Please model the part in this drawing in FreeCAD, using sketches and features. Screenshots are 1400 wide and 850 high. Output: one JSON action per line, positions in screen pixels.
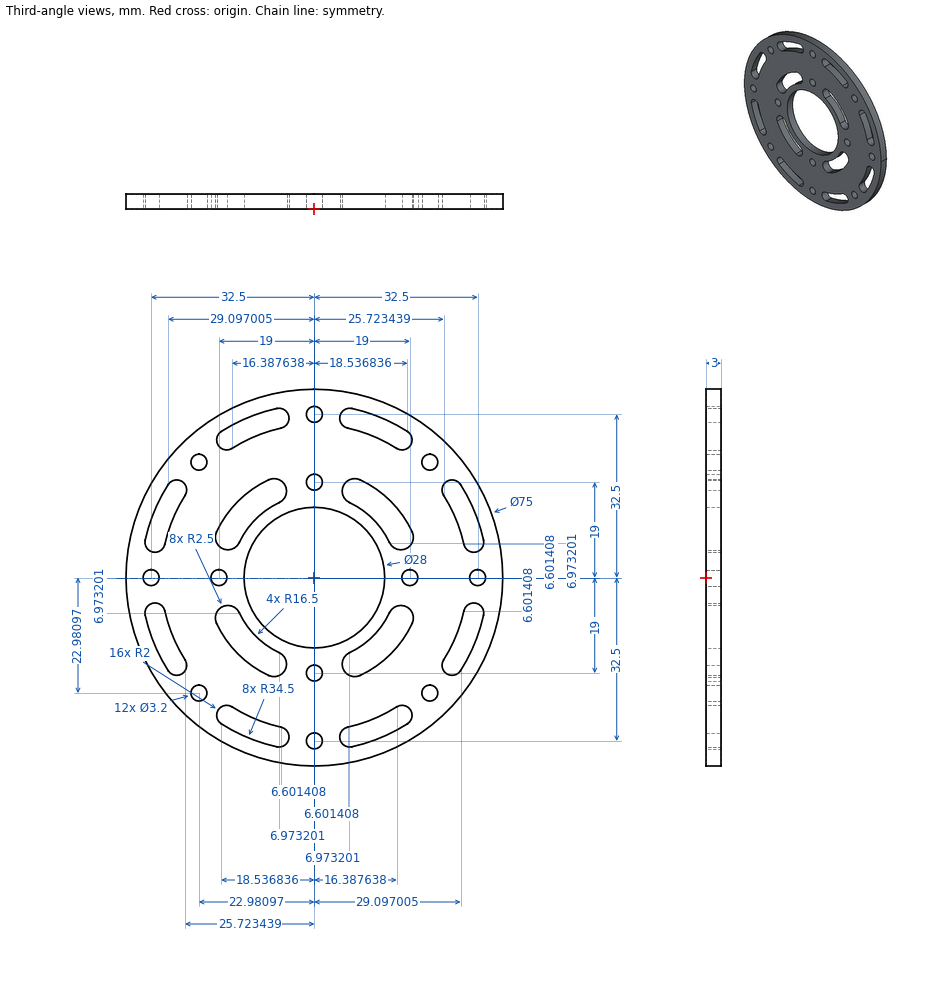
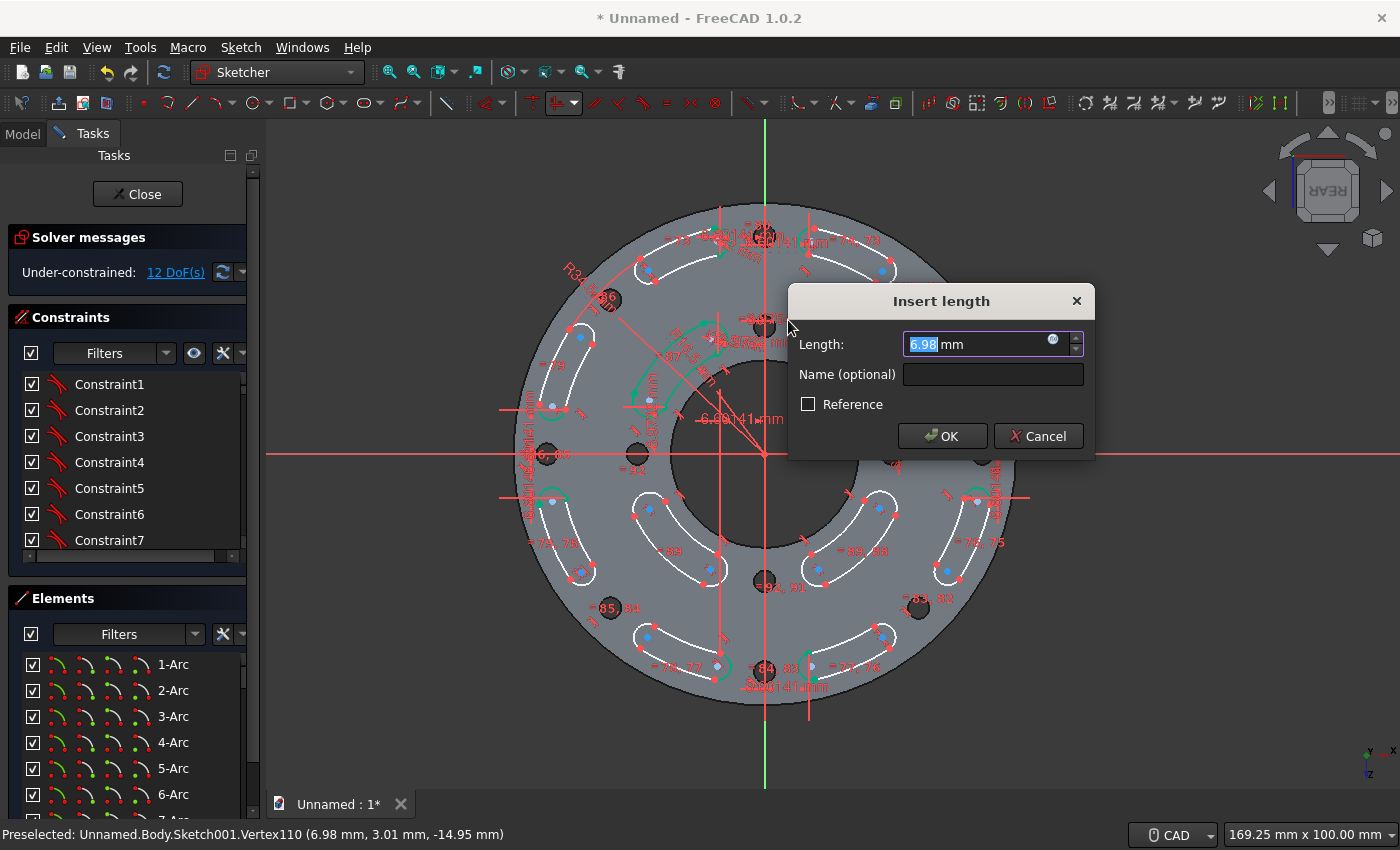
{"action": "type", "text": "6.973201"}
{"action": "key", "text": "Return"}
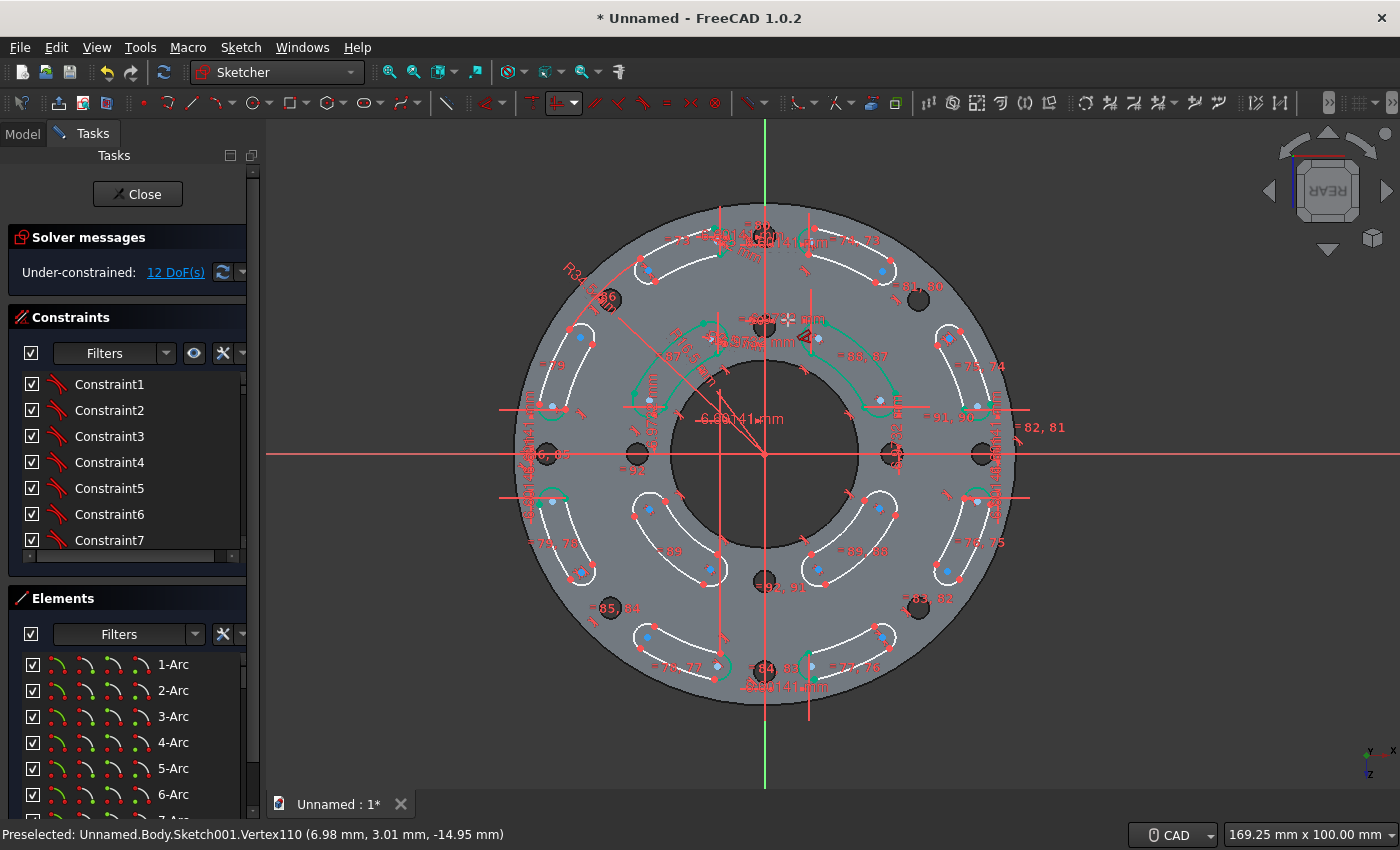
{"action": "left_click", "coordinate": [811, 554]}
{"action": "left_click", "coordinate": [788, 588]}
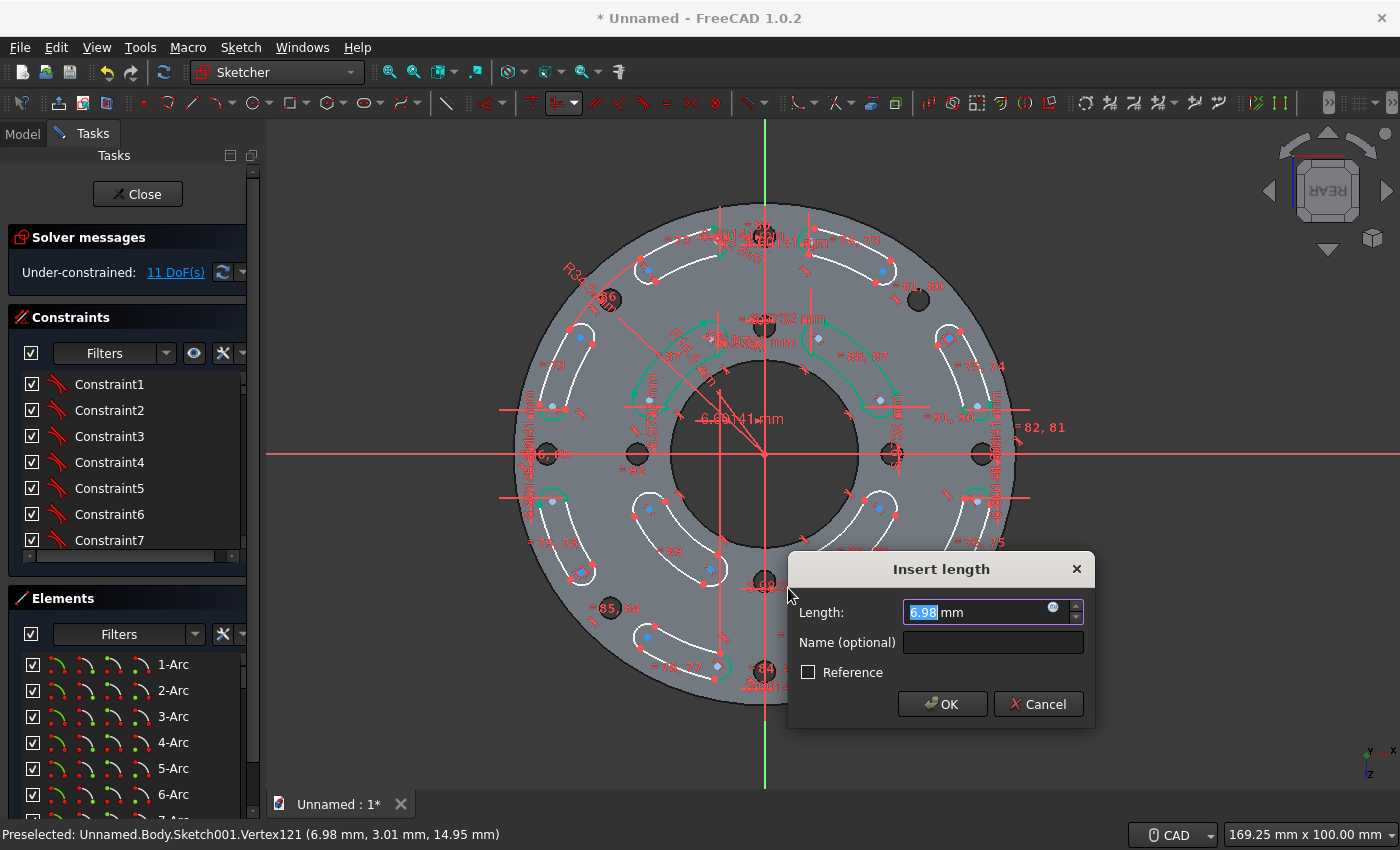
{"action": "type", "text": "6.973201"}
{"action": "key", "text": "Return"}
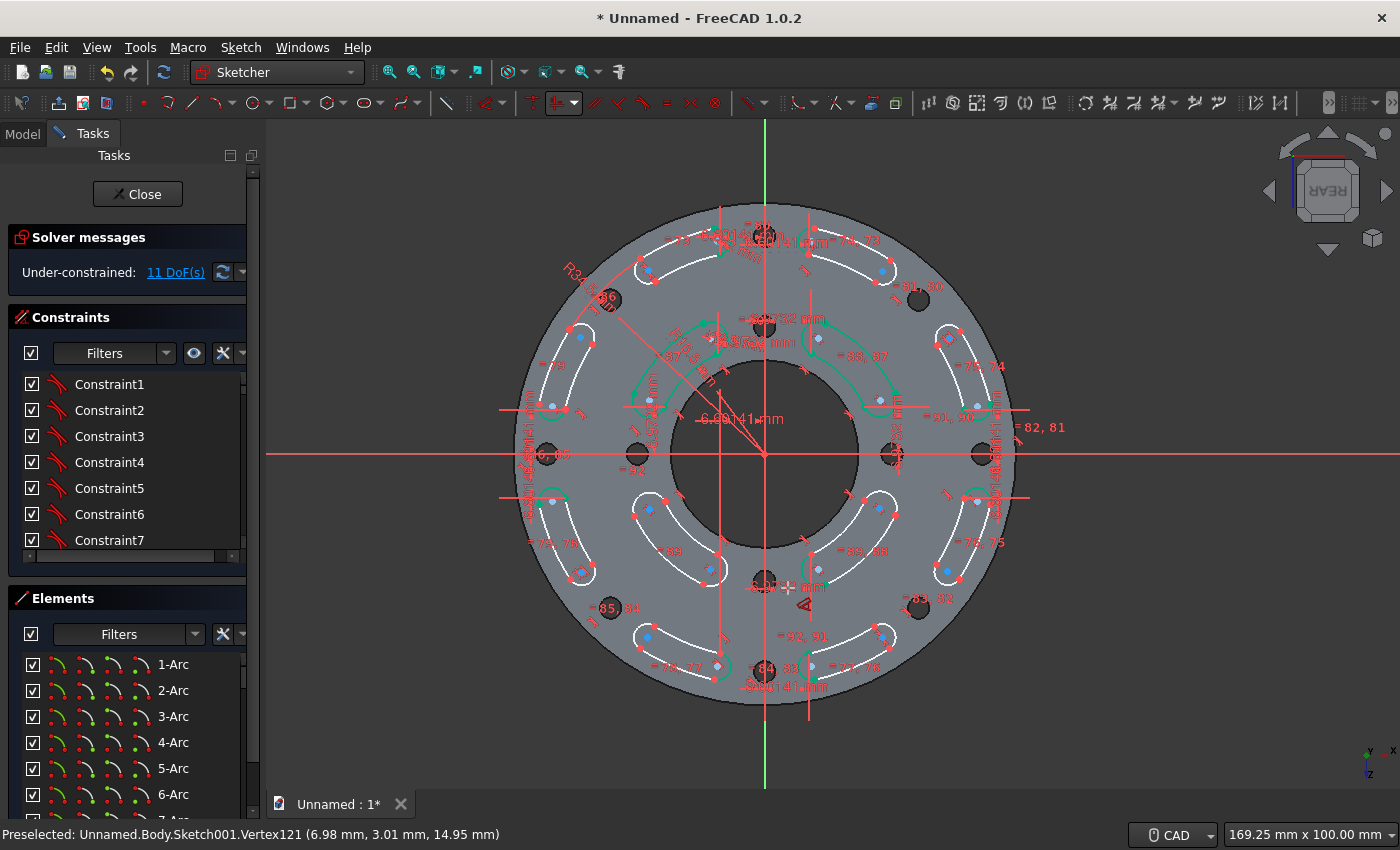
{"action": "left_click", "coordinate": [865, 501]}
{"action": "left_click", "coordinate": [899, 478]}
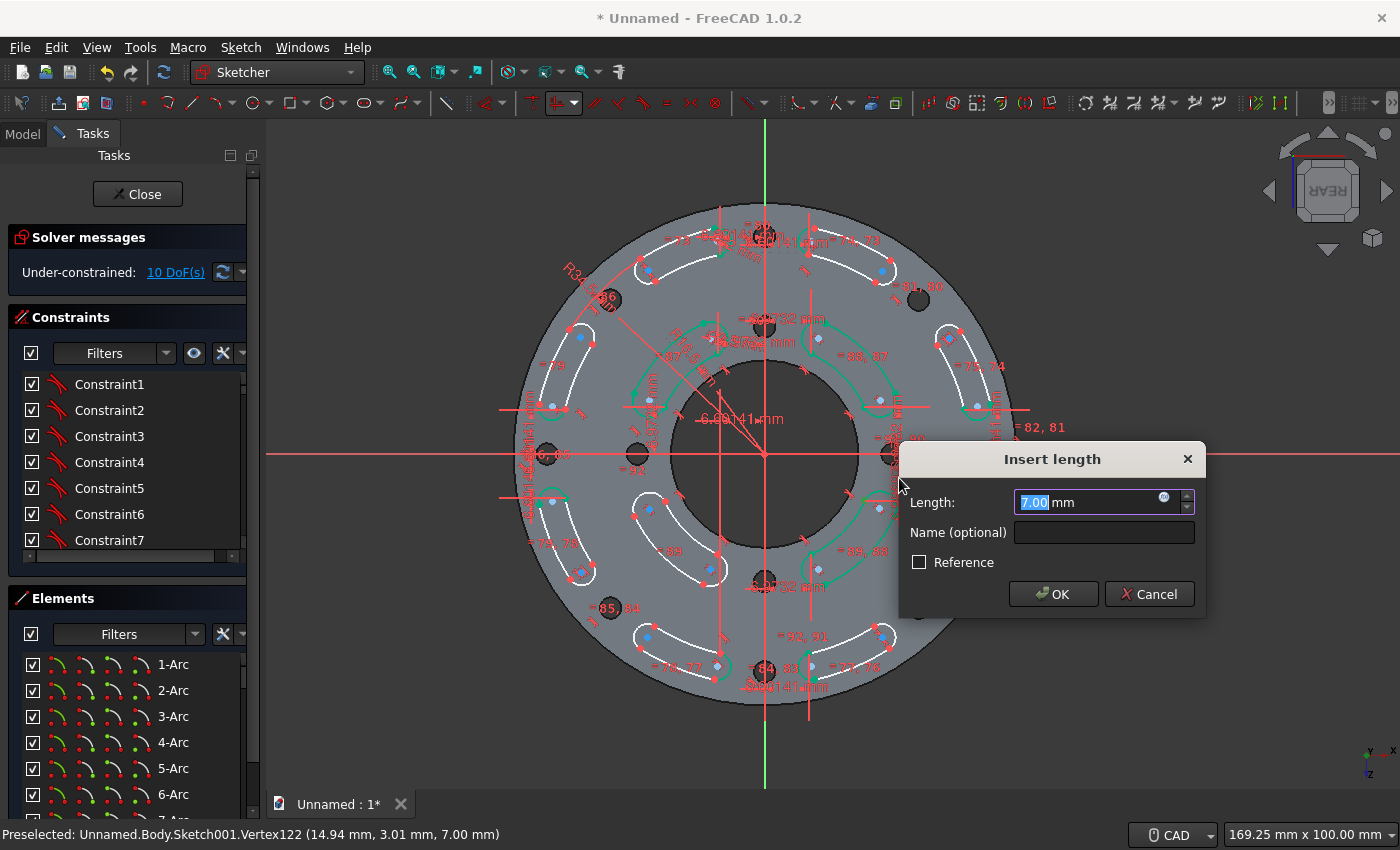
{"action": "type", "text": "6.973201"}
{"action": "key", "text": "Return"}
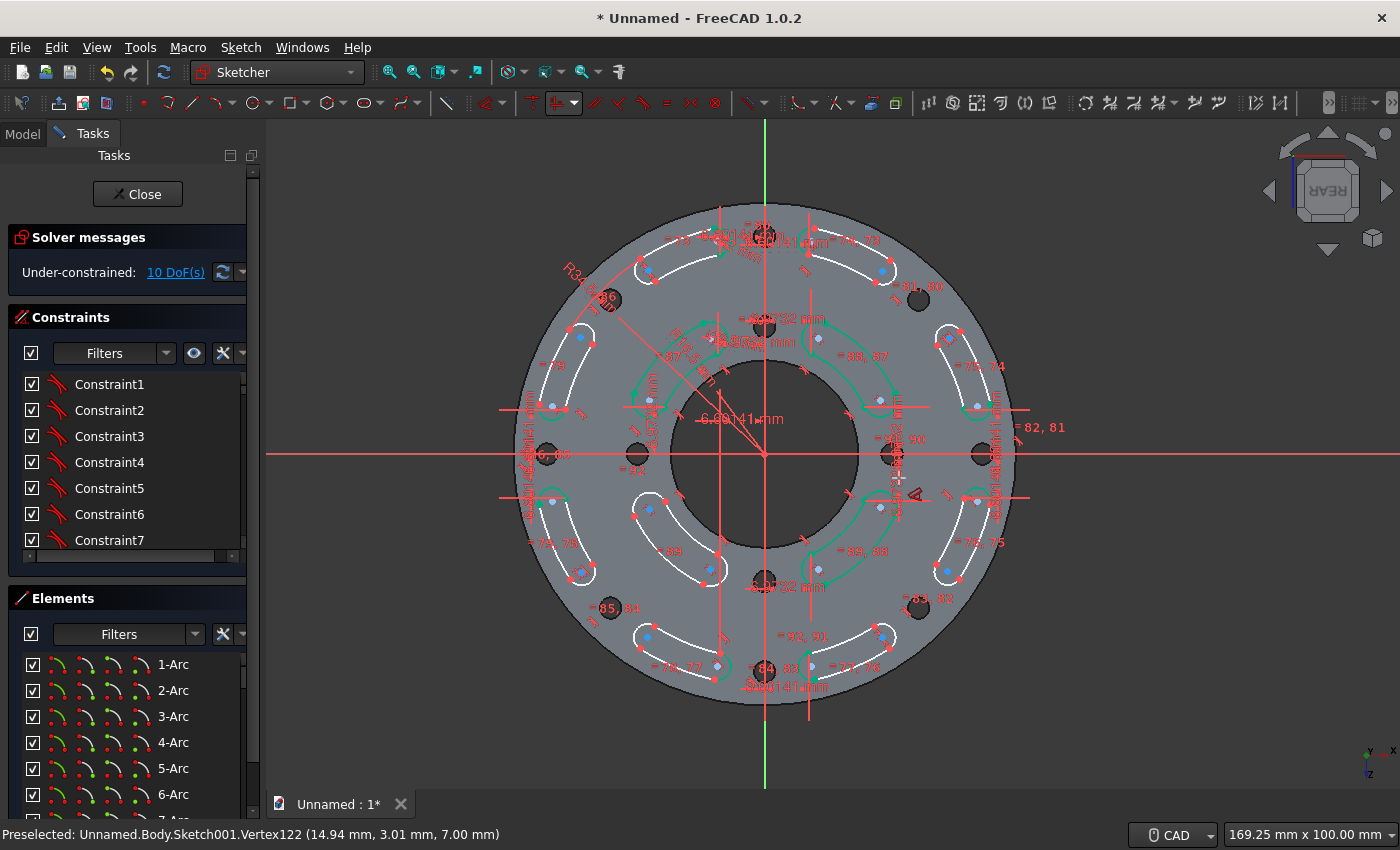
{"action": "left_click", "coordinate": [665, 502]}
{"action": "left_click", "coordinate": [631, 478]}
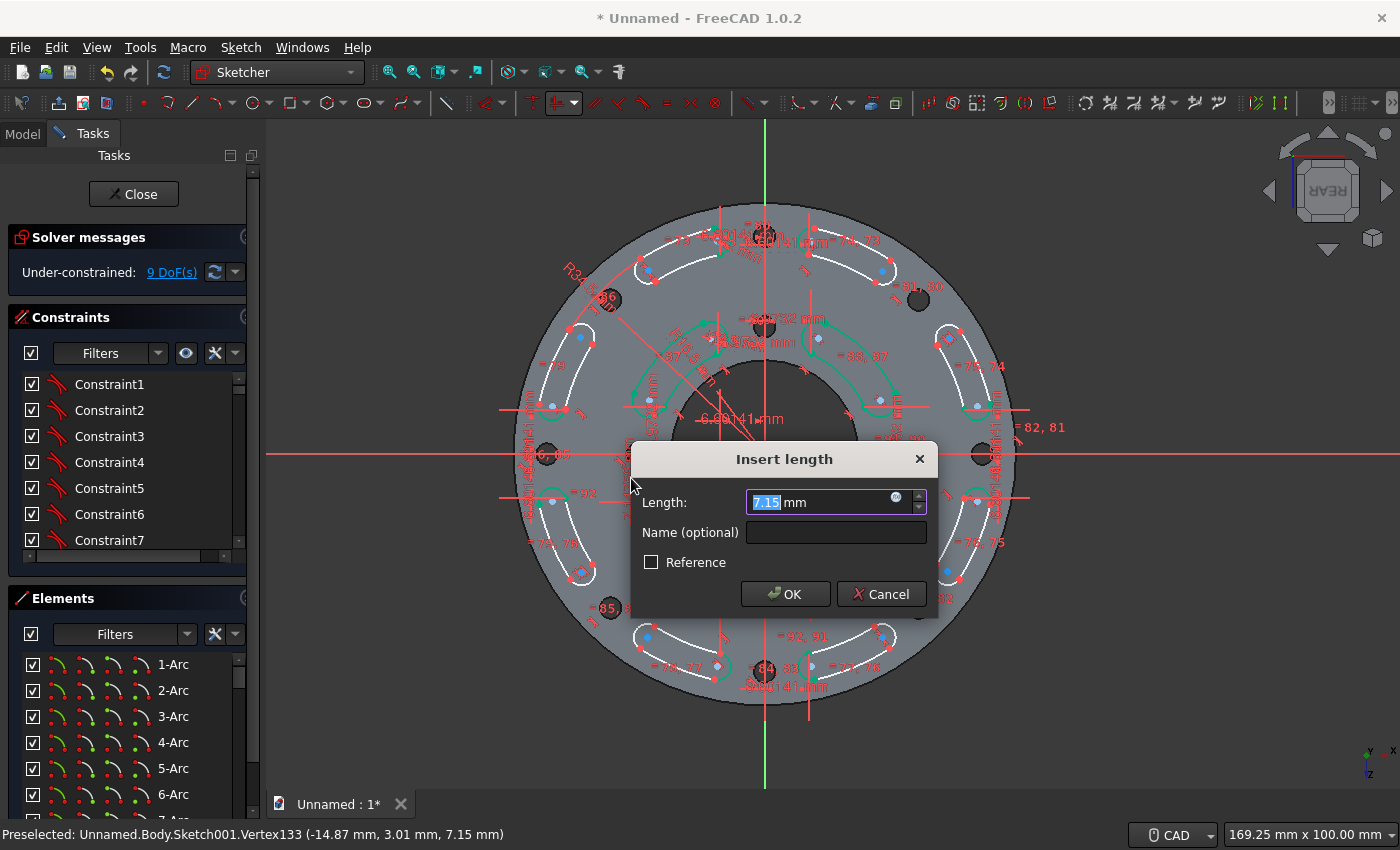
{"action": "type", "text": "6.973201"}
{"action": "key", "text": "Return"}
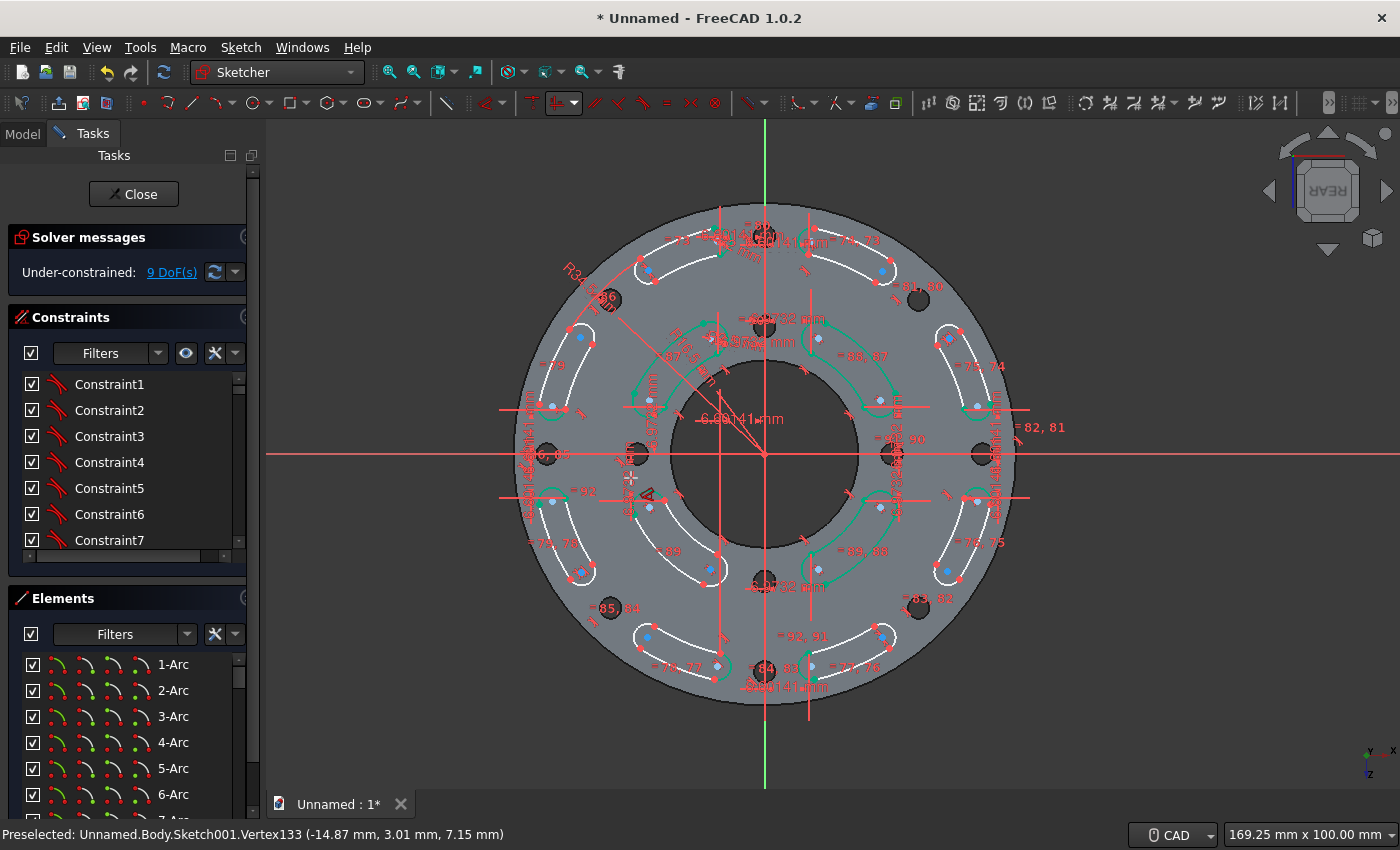
{"action": "left_click", "coordinate": [718, 554]}
{"action": "left_click", "coordinate": [741, 612]}